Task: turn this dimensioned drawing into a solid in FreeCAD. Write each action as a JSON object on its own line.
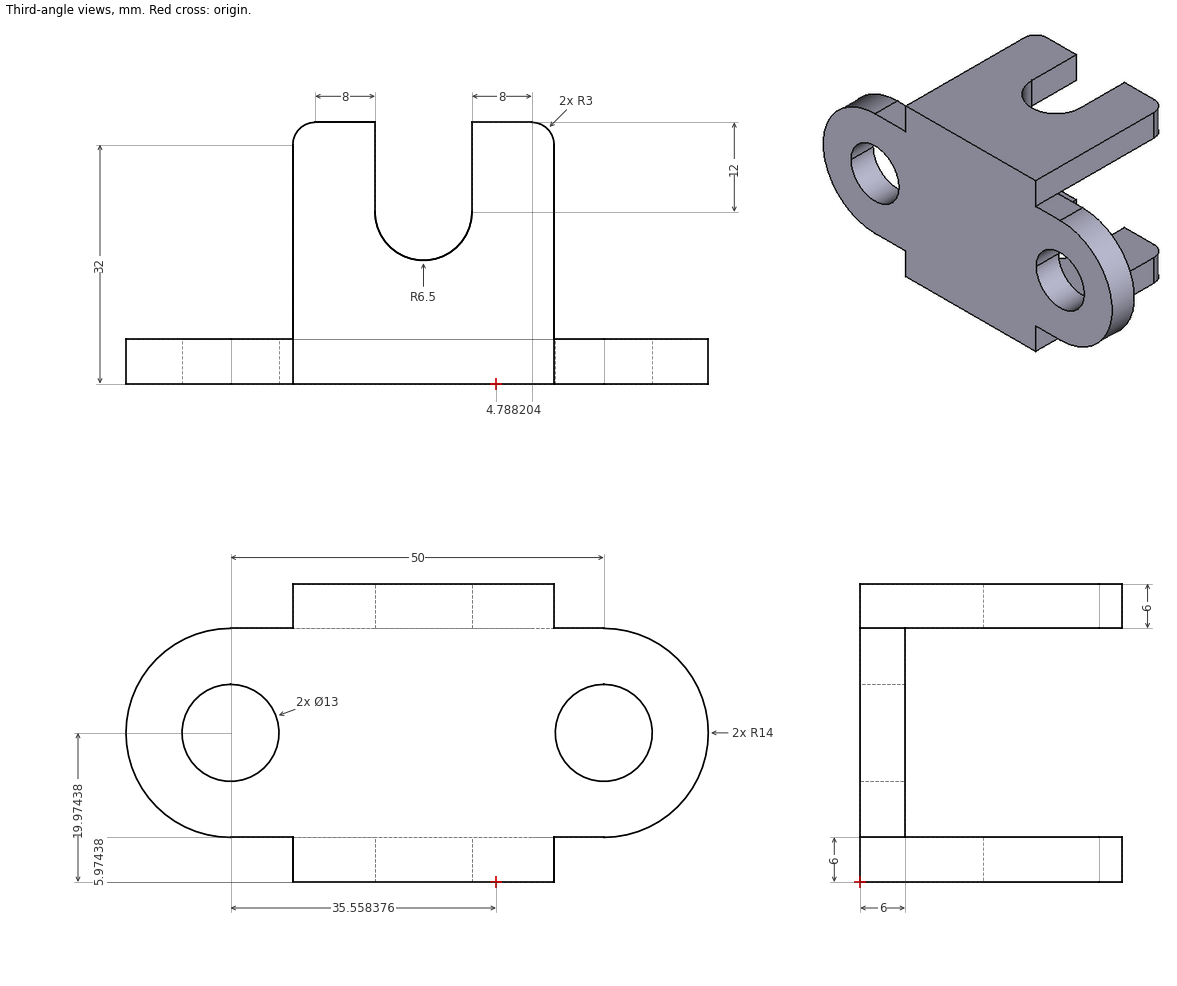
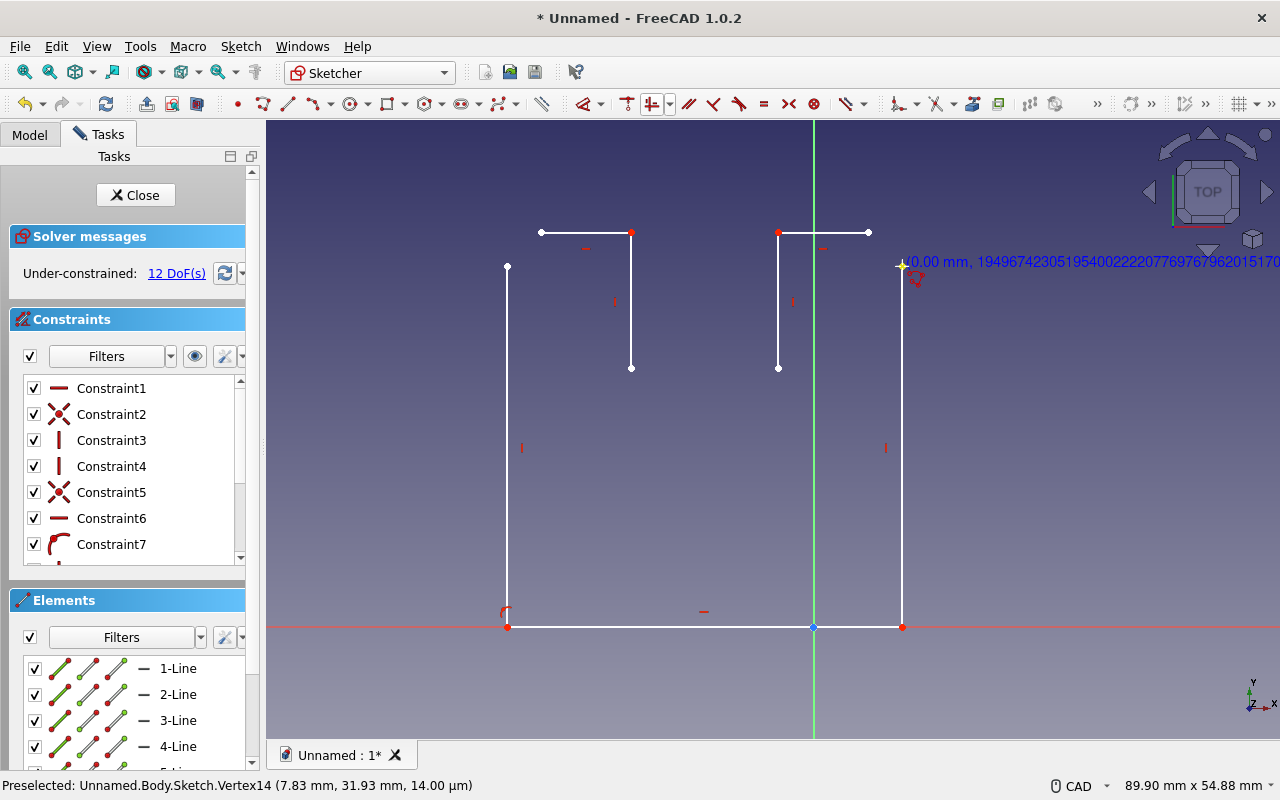
{"action": "left_click", "coordinate": [312, 104]}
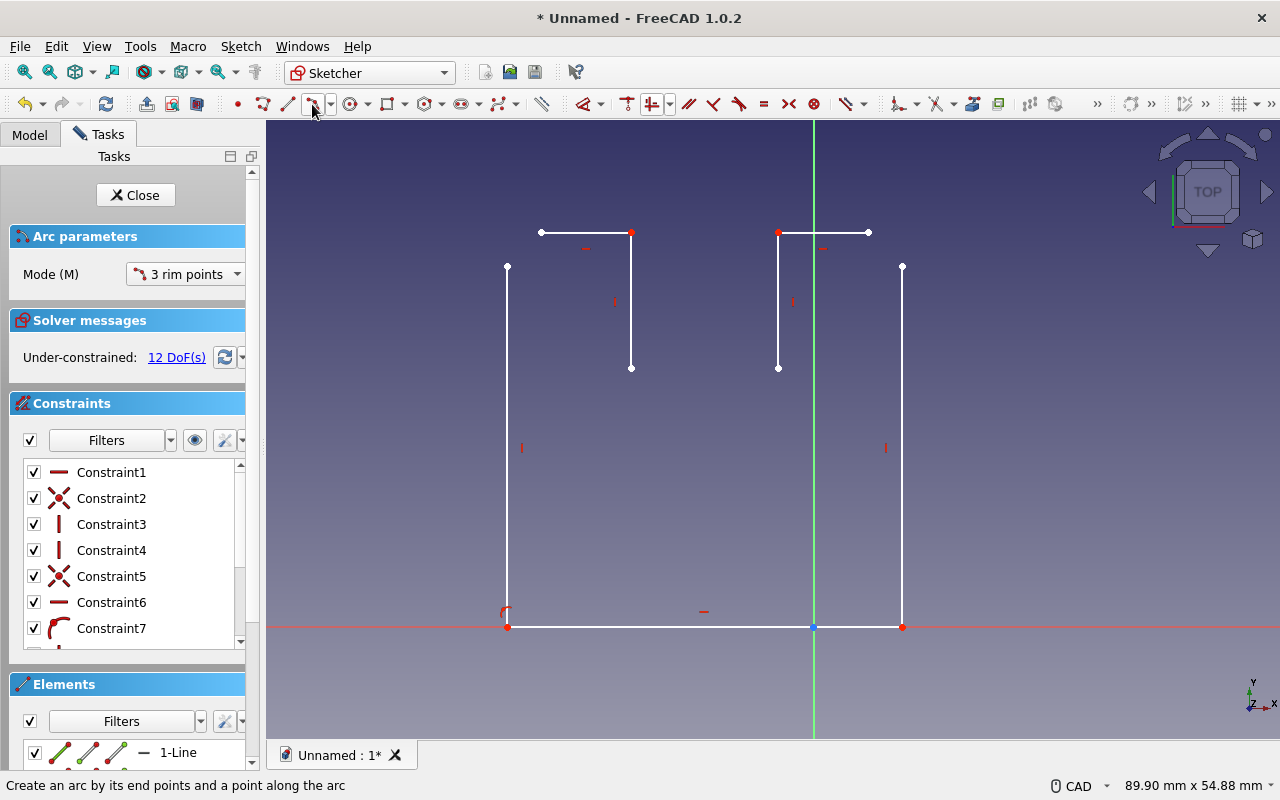
{"action": "left_click", "coordinate": [778, 369]}
{"action": "left_click", "coordinate": [631, 369]}
{"action": "left_click", "coordinate": [704, 441]}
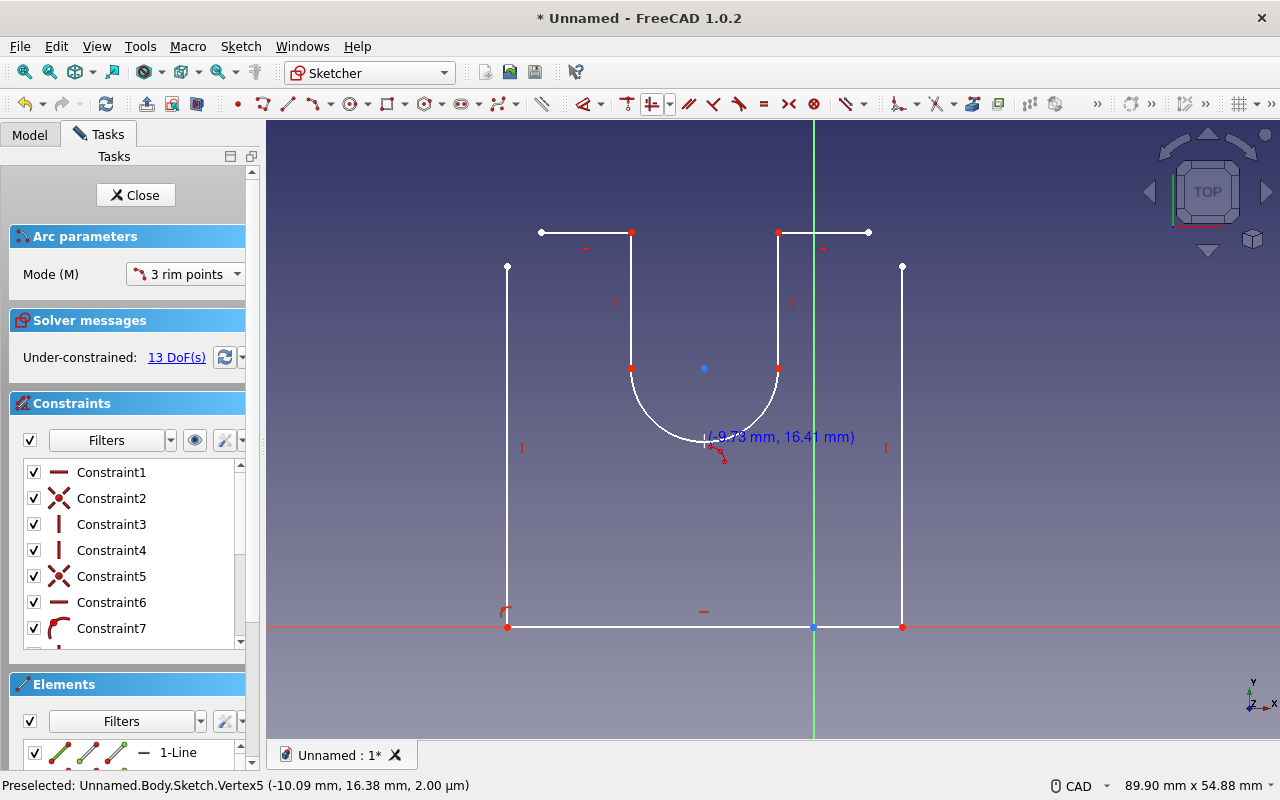
{"action": "left_click", "coordinate": [541, 233]}
{"action": "left_click", "coordinate": [507, 267]}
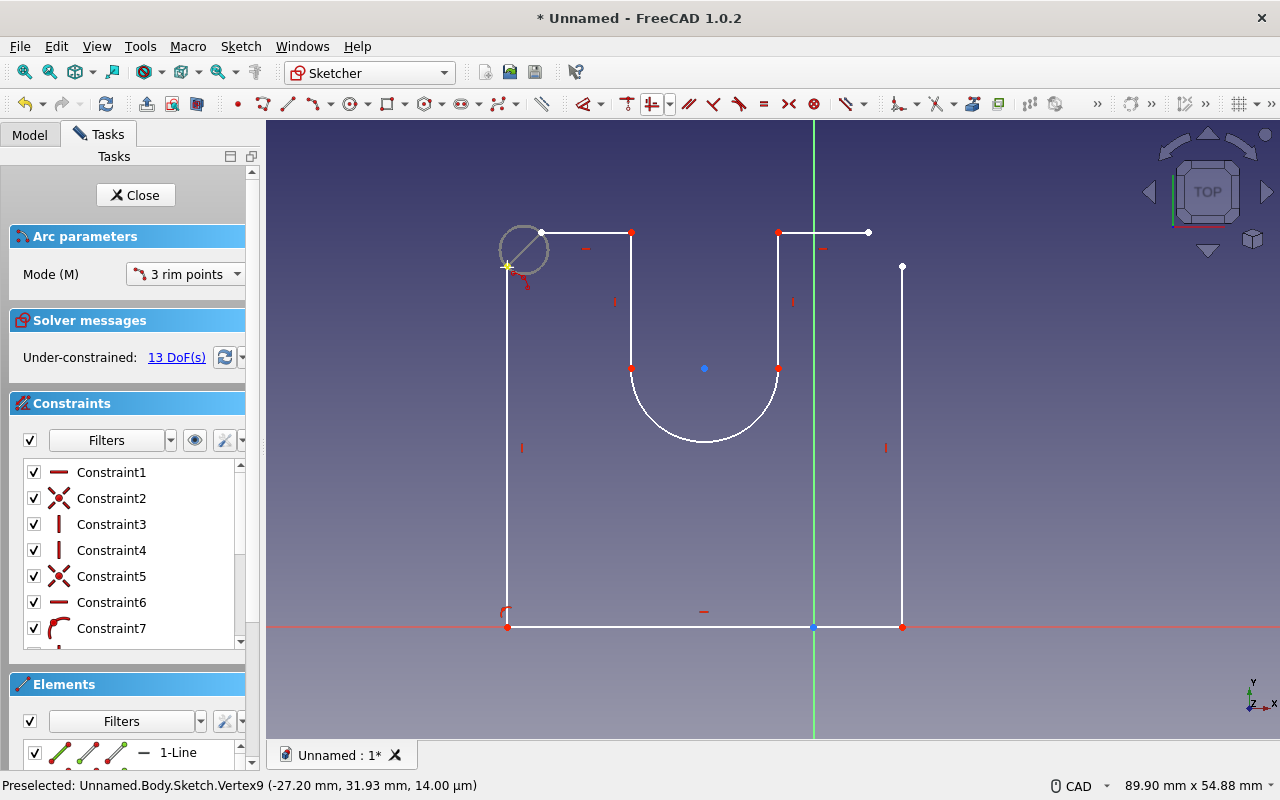
{"action": "scroll", "coordinate": [517, 242], "scroll_direction": "up", "scroll_amount": 3}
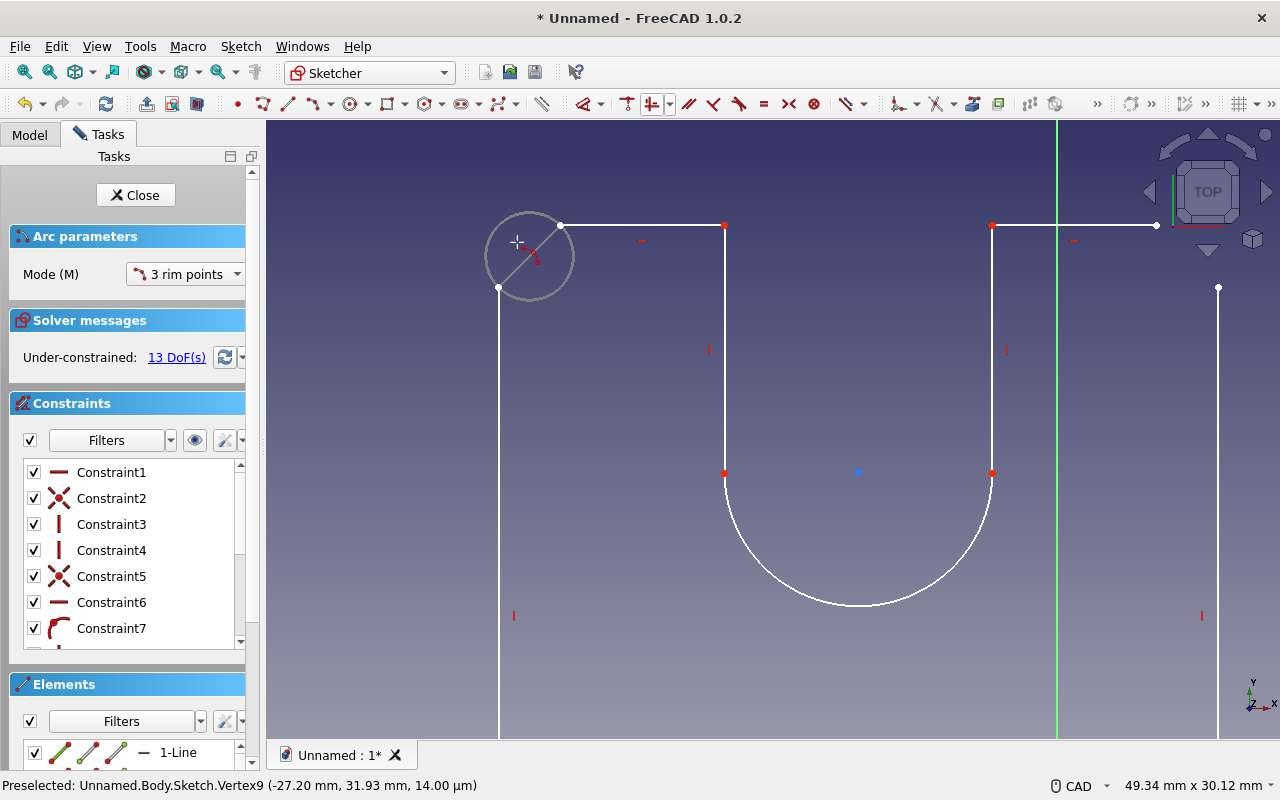
{"action": "left_click", "coordinate": [516, 242]}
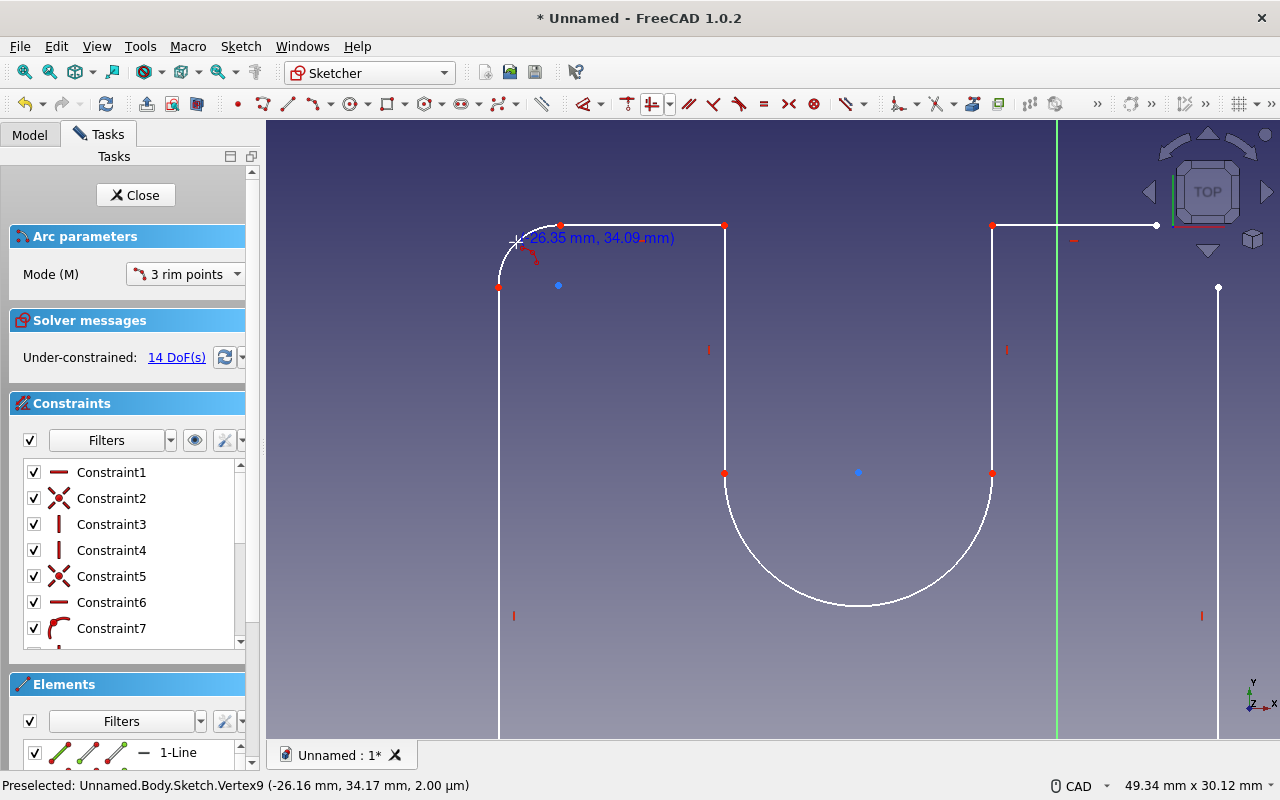
{"action": "scroll", "coordinate": [518, 242], "scroll_direction": "down", "scroll_amount": 3}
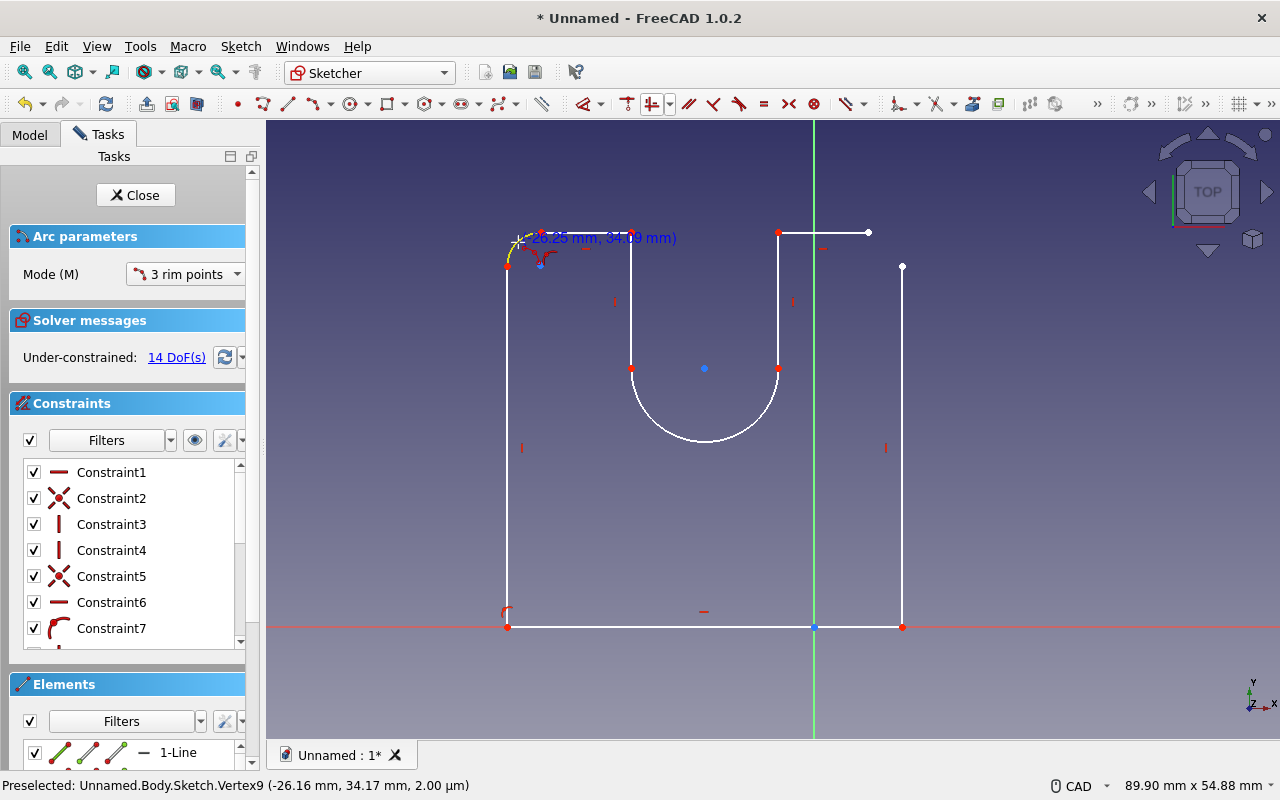
{"action": "left_click", "coordinate": [902, 267]}
{"action": "left_click", "coordinate": [868, 233]}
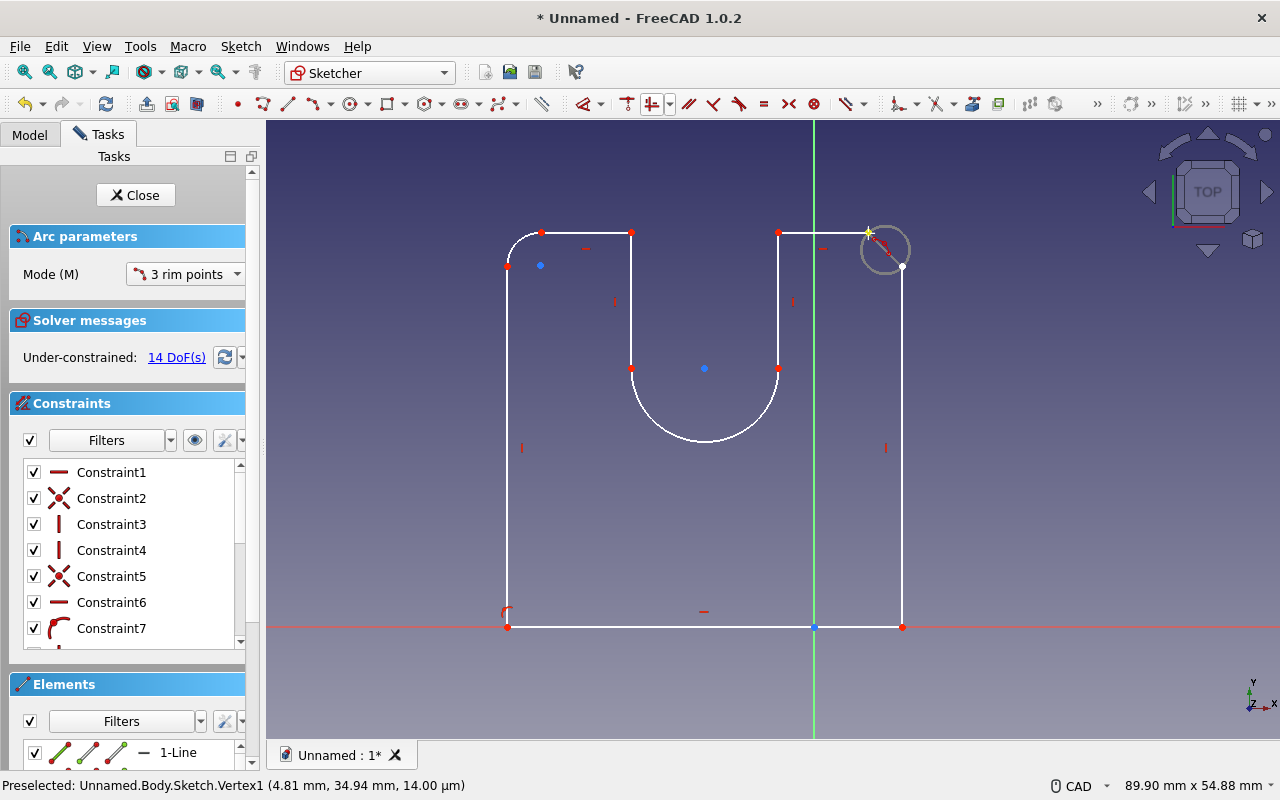
{"action": "scroll", "coordinate": [892, 242], "scroll_direction": "up", "scroll_amount": 3}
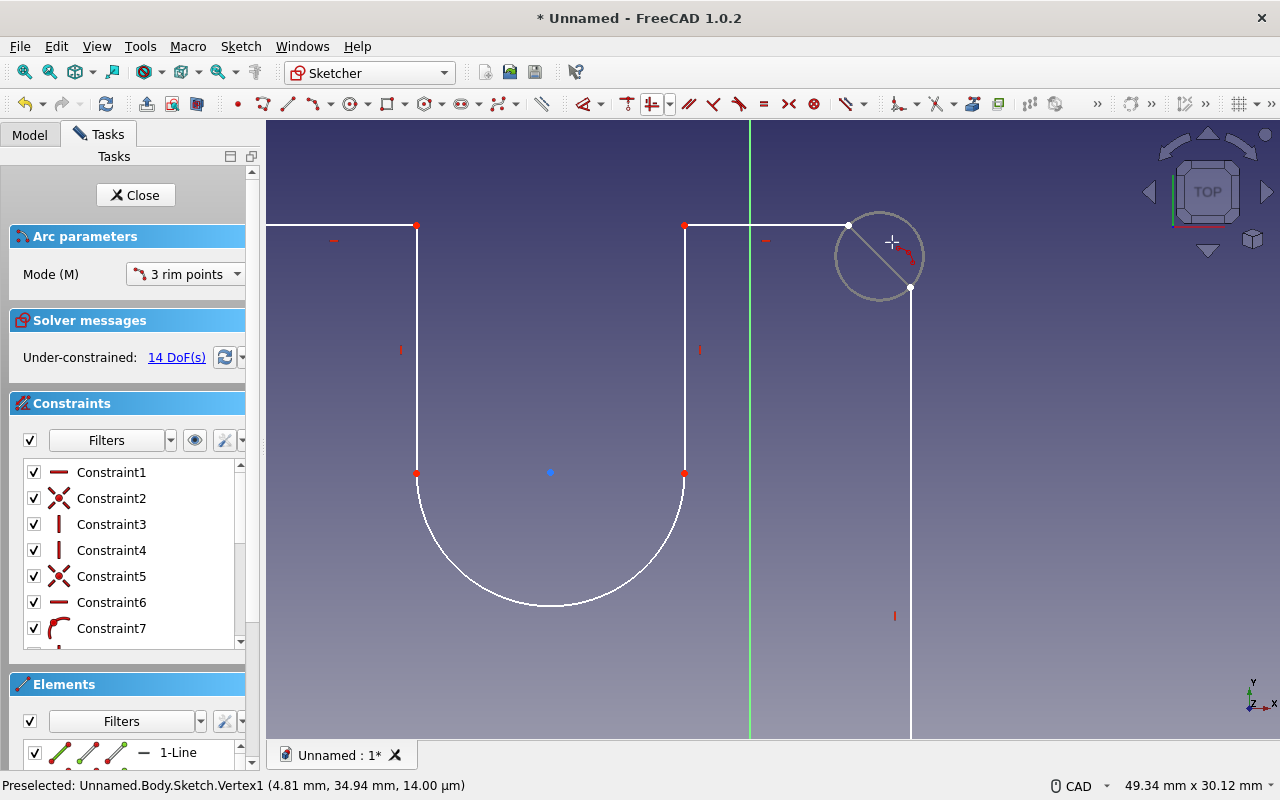
{"action": "left_click", "coordinate": [892, 242]}
{"action": "key", "text": "Escape"}